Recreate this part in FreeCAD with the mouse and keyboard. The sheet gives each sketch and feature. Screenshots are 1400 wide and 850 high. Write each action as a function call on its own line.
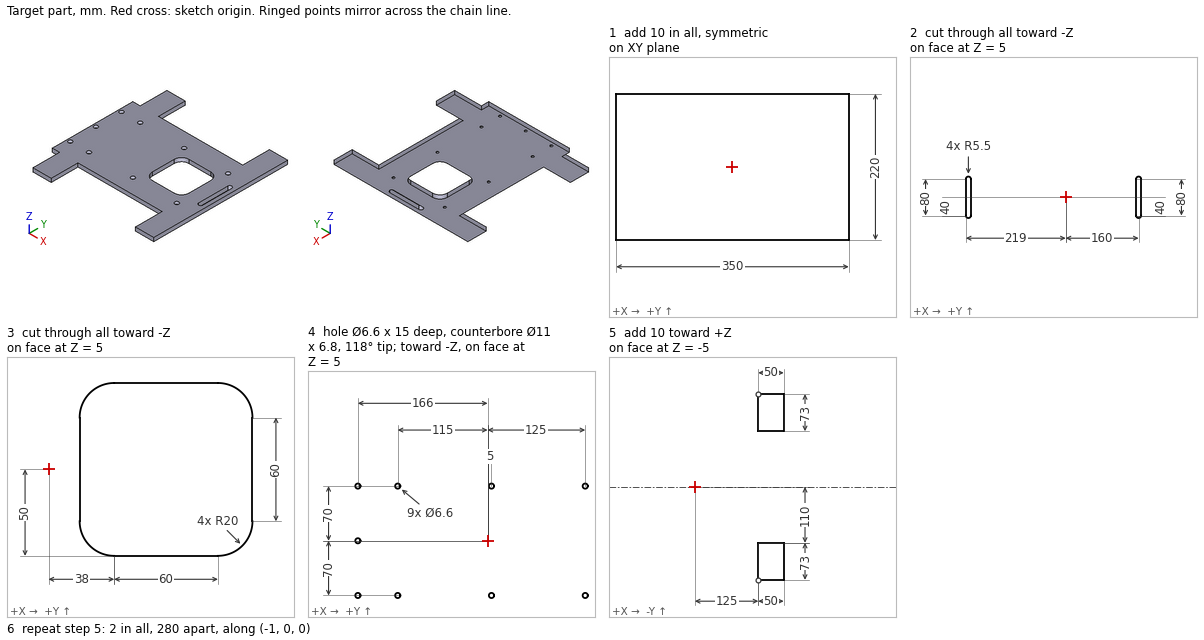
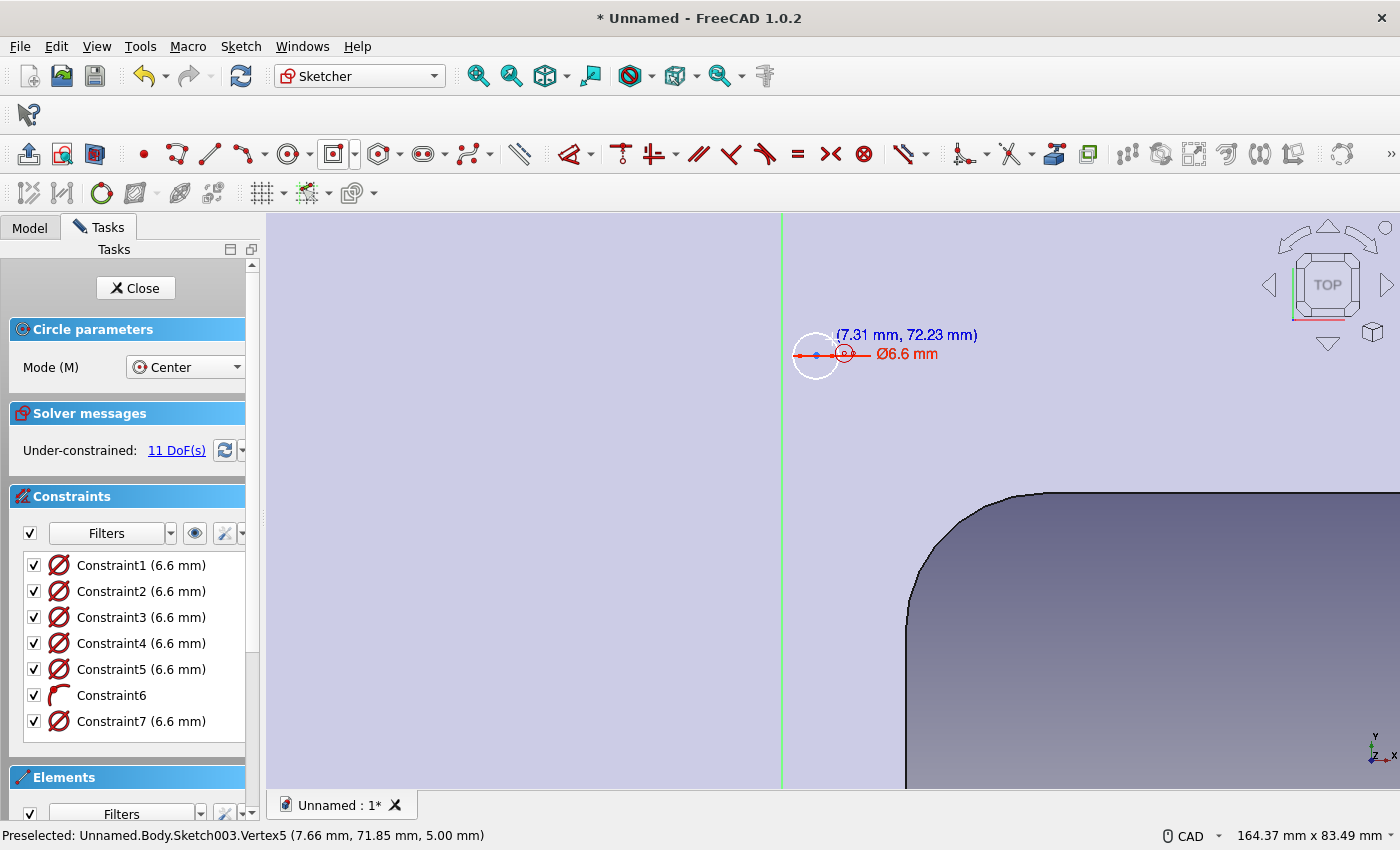
scroll(818, 356, down, 6)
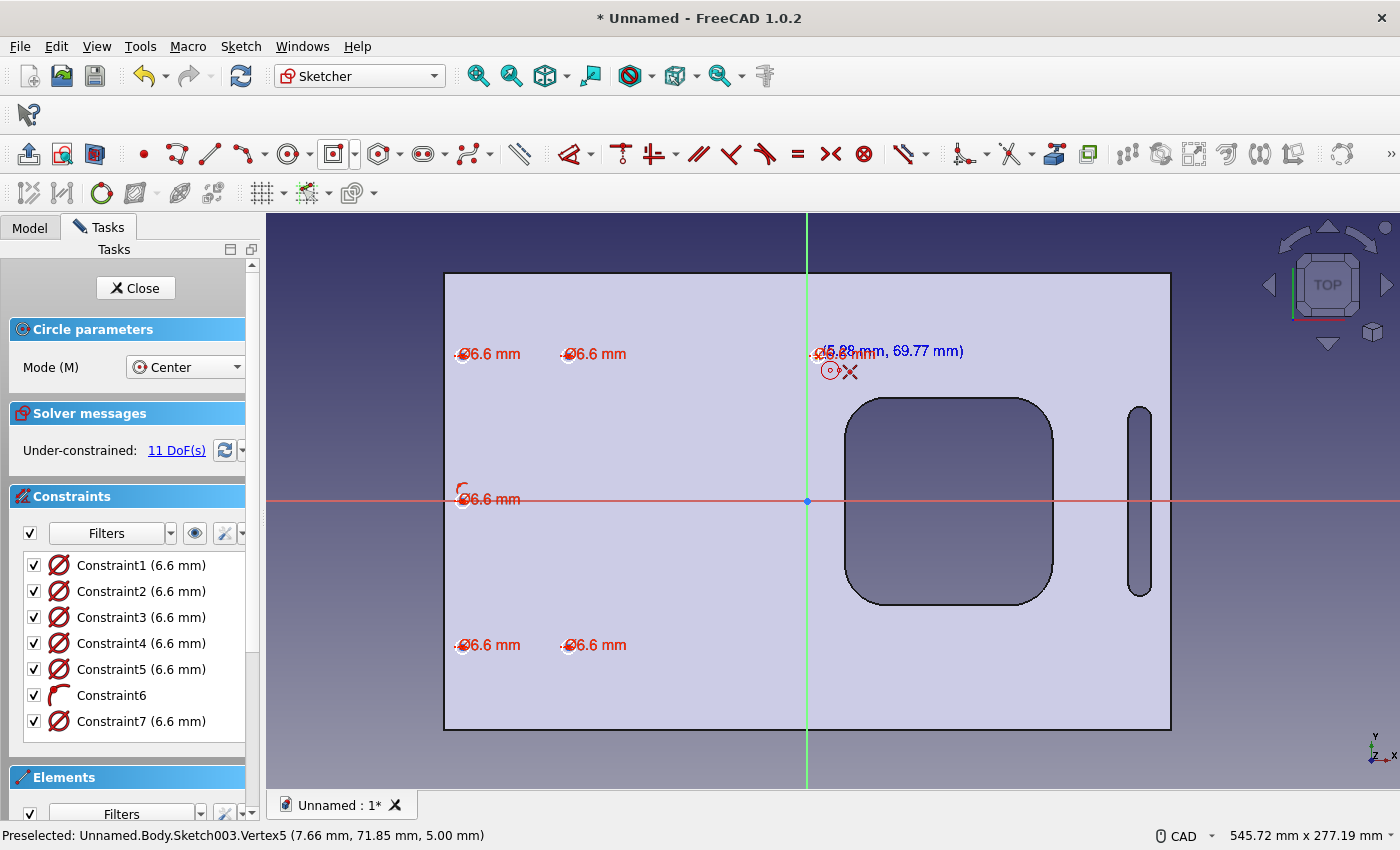
scroll(1067, 356, up, 6)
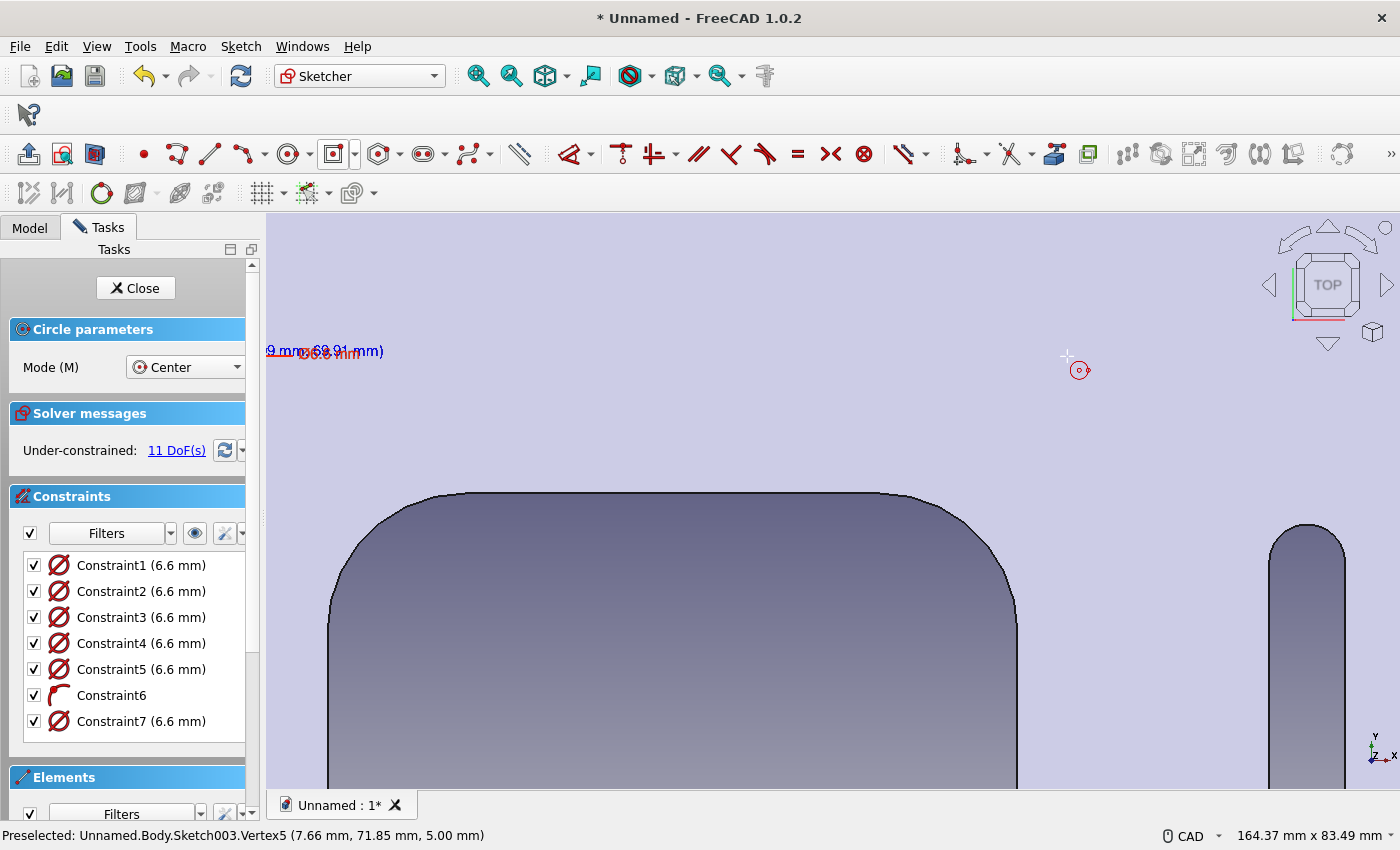
click(1066, 355)
move(1082, 339)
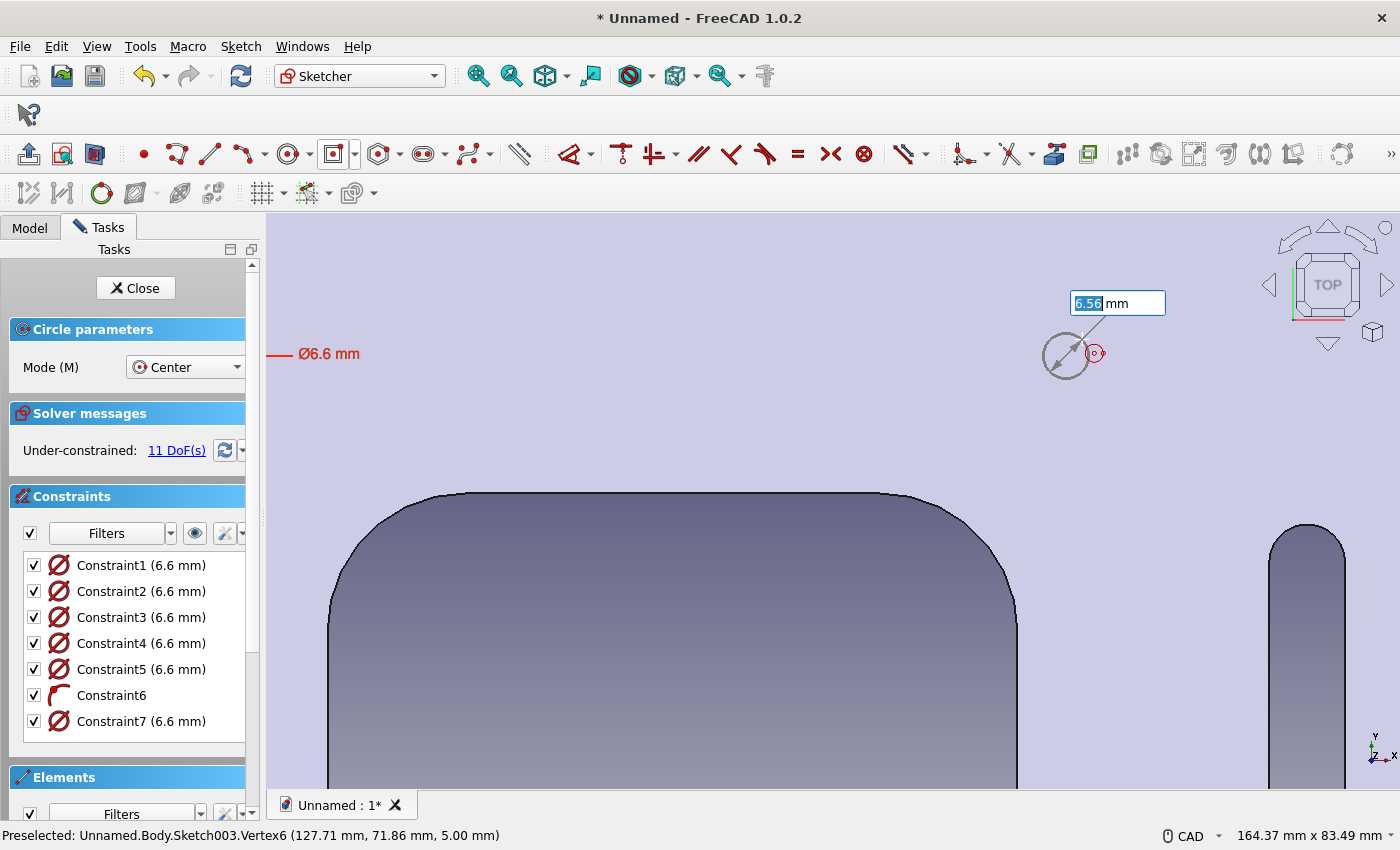
text(6.6)
key(Return)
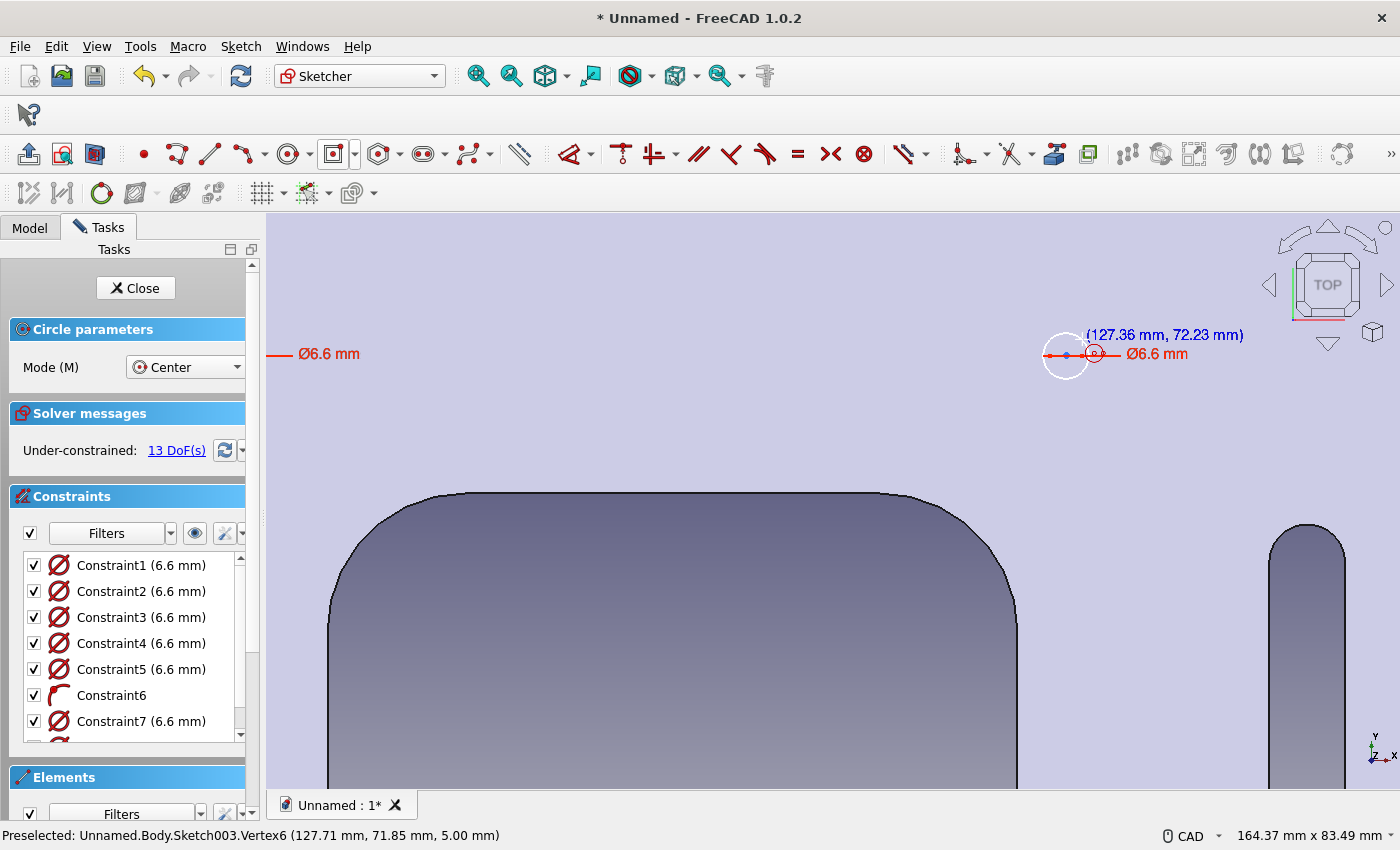
scroll(1067, 356, down, 6)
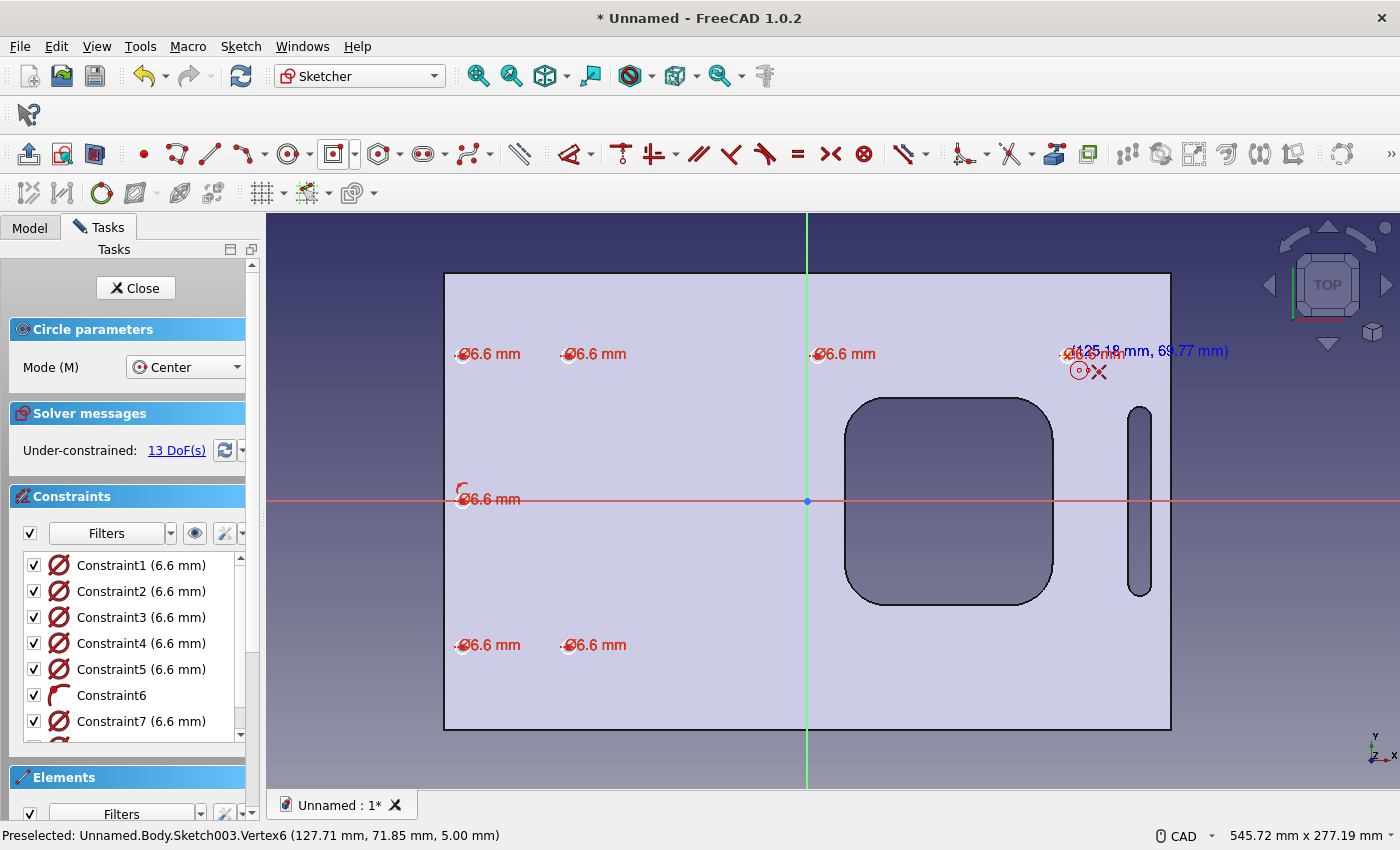
scroll(1067, 647, up, 6)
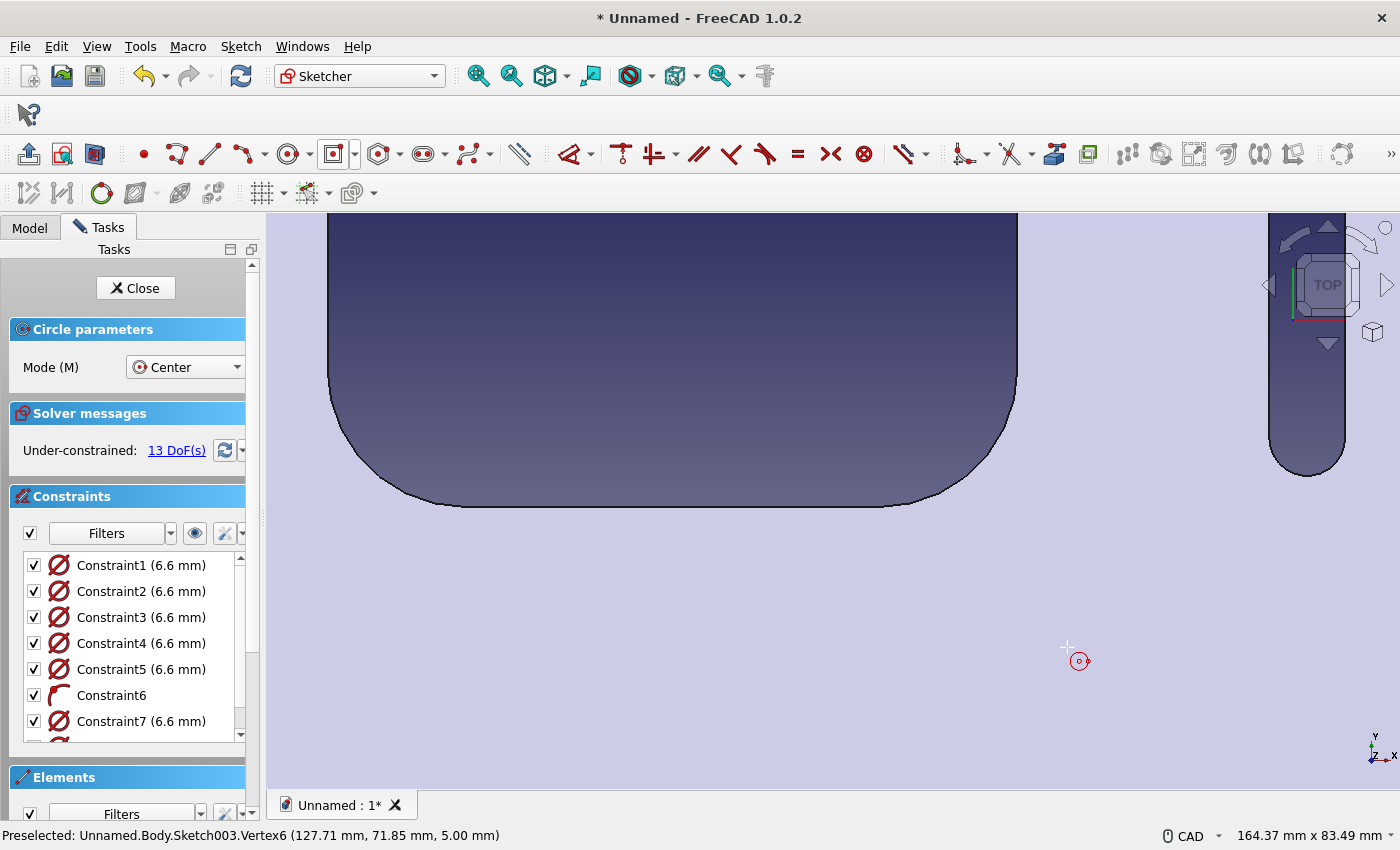
click(1066, 645)
move(1082, 629)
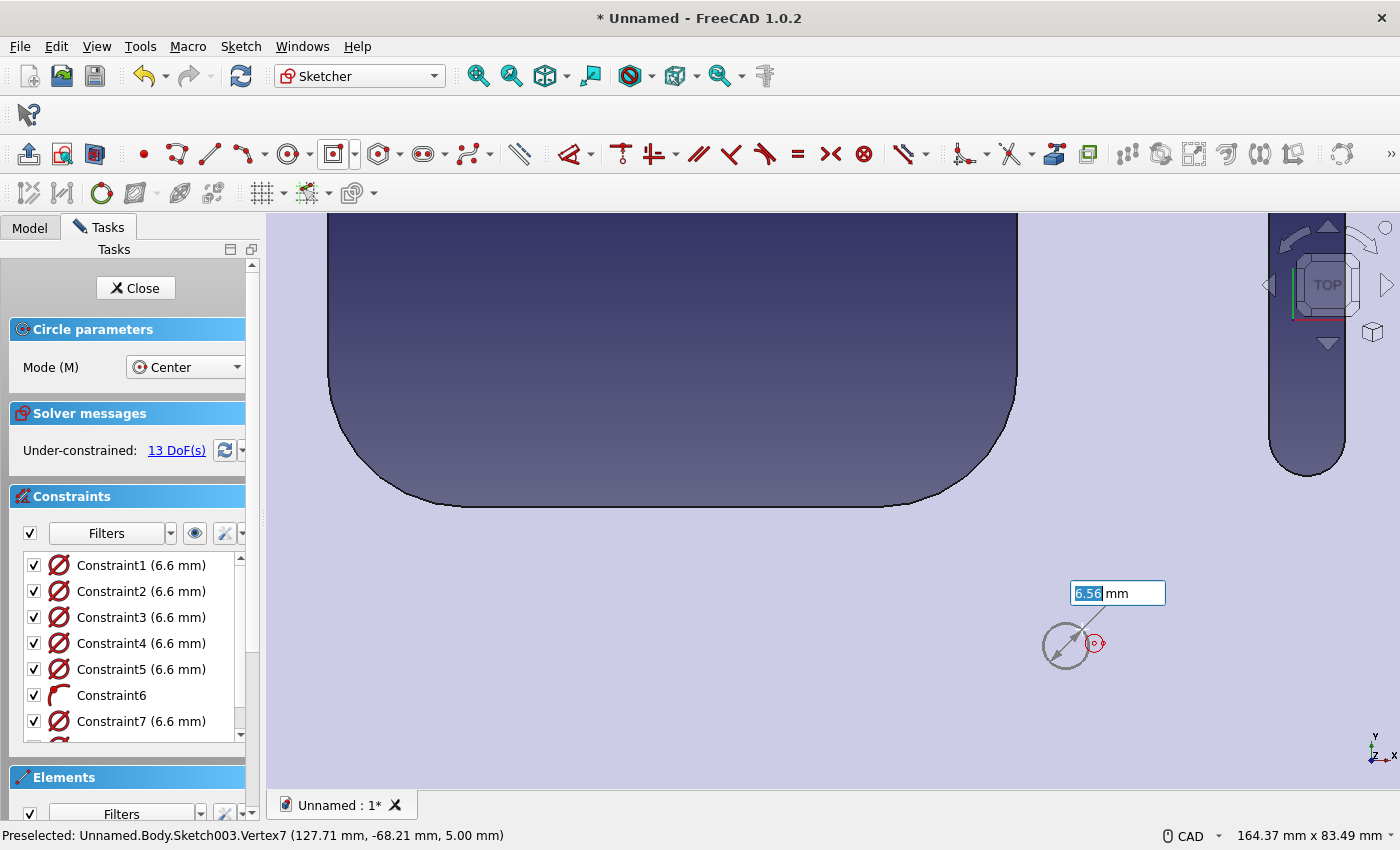
text(6.6)
key(Return)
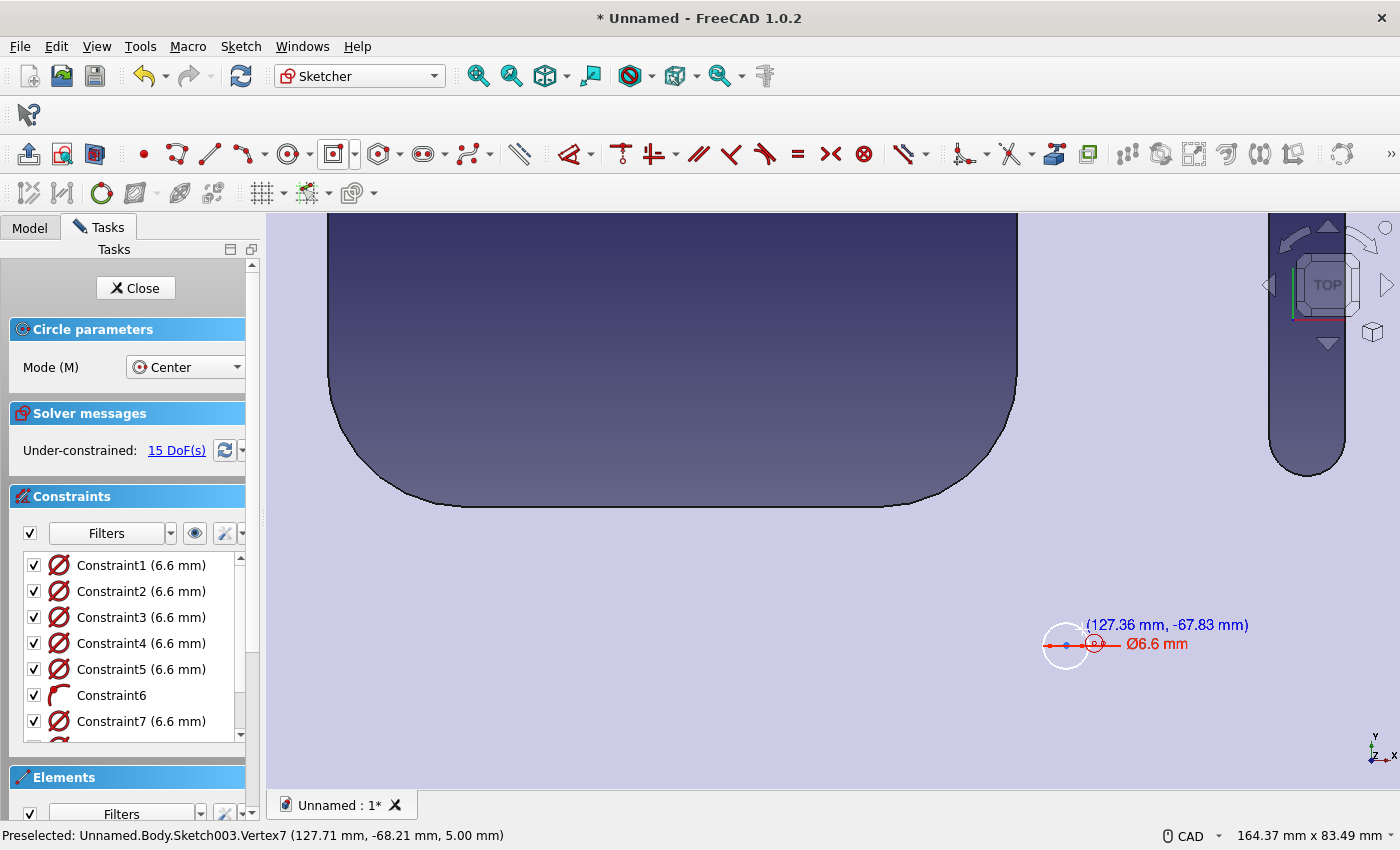
scroll(1067, 647, down, 6)